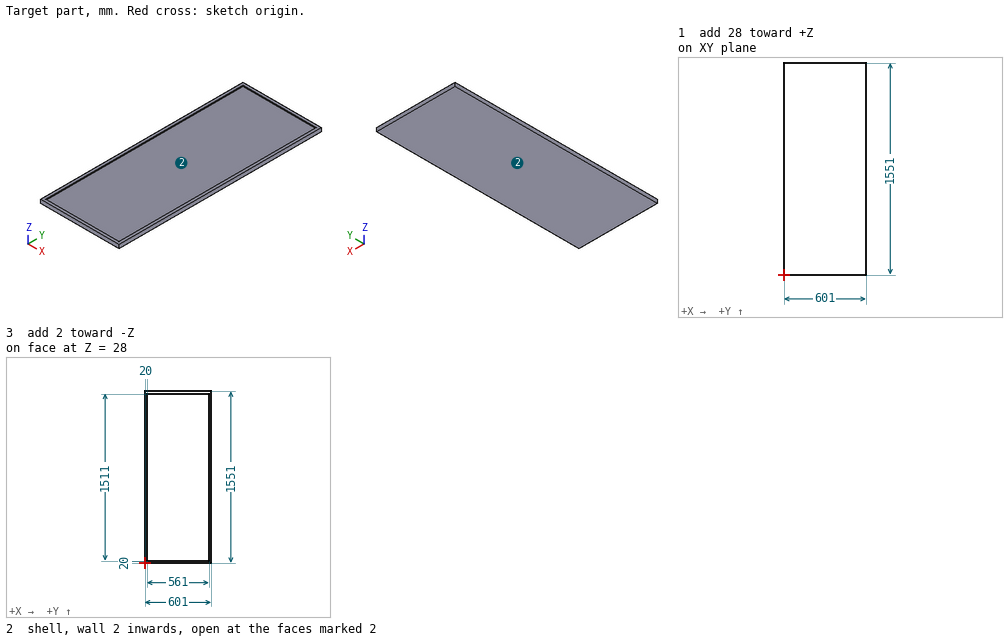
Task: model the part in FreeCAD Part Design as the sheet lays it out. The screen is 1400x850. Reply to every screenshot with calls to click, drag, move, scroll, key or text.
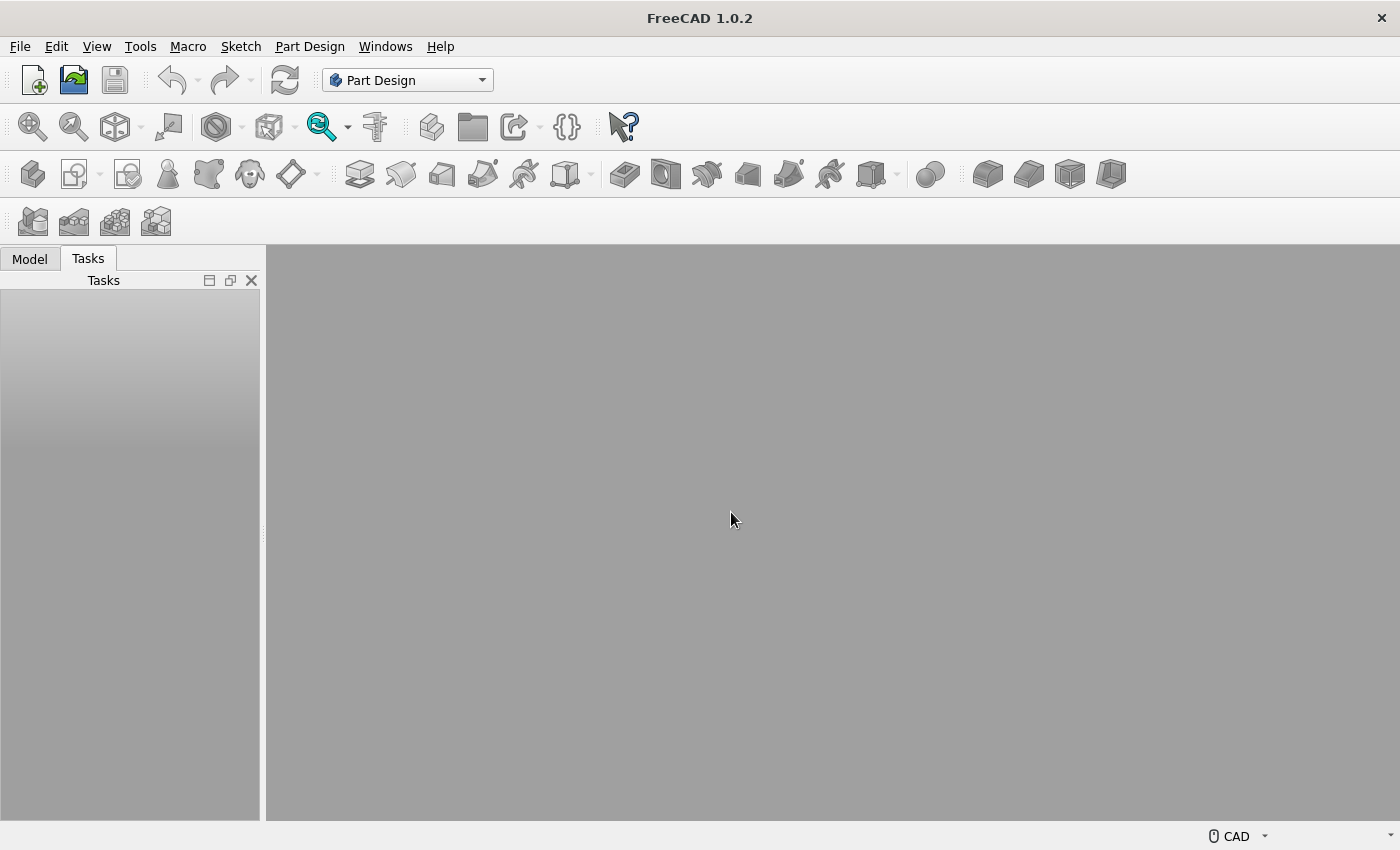
click(33, 80)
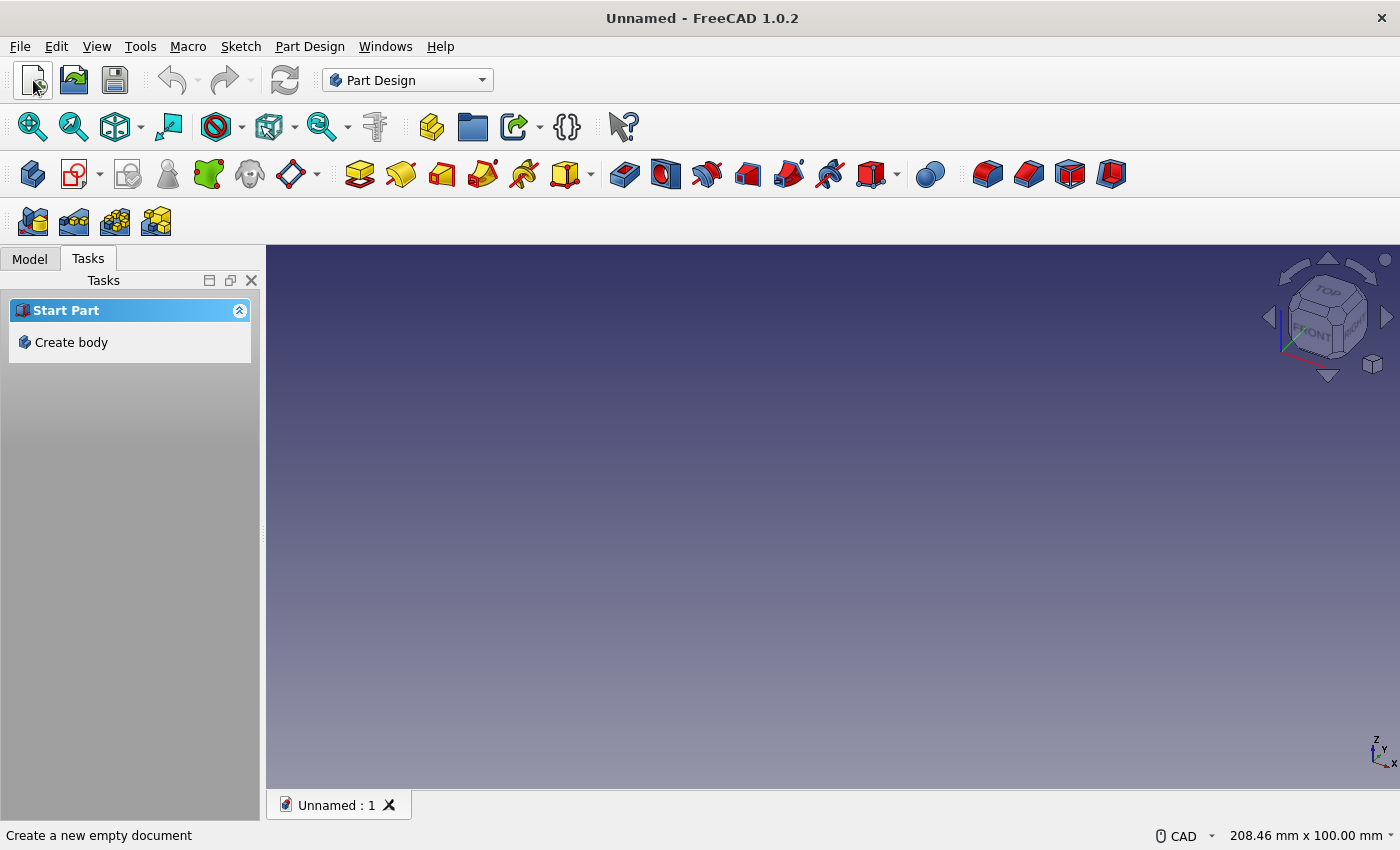
click(74, 174)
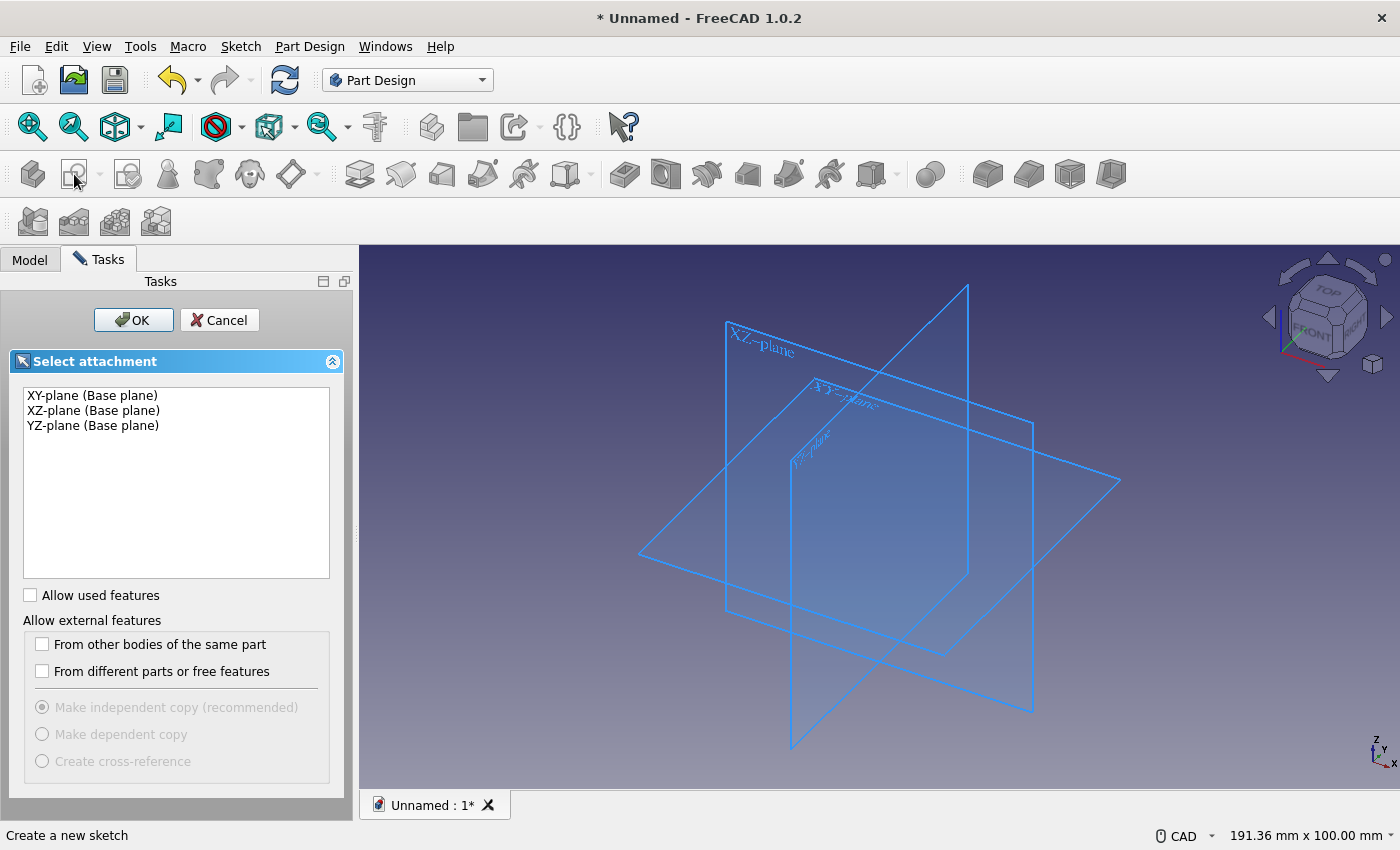
click(84, 396)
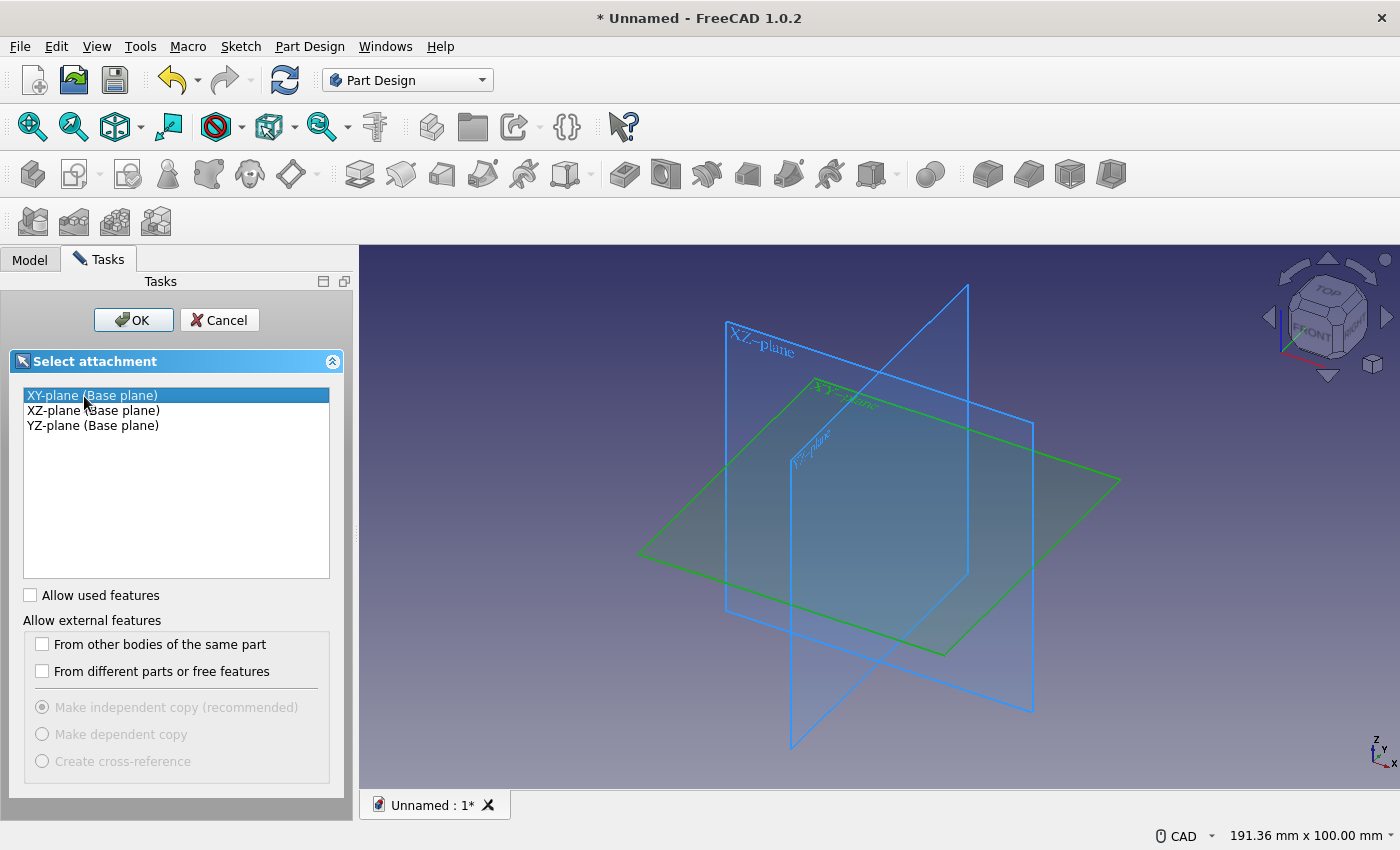
click(134, 320)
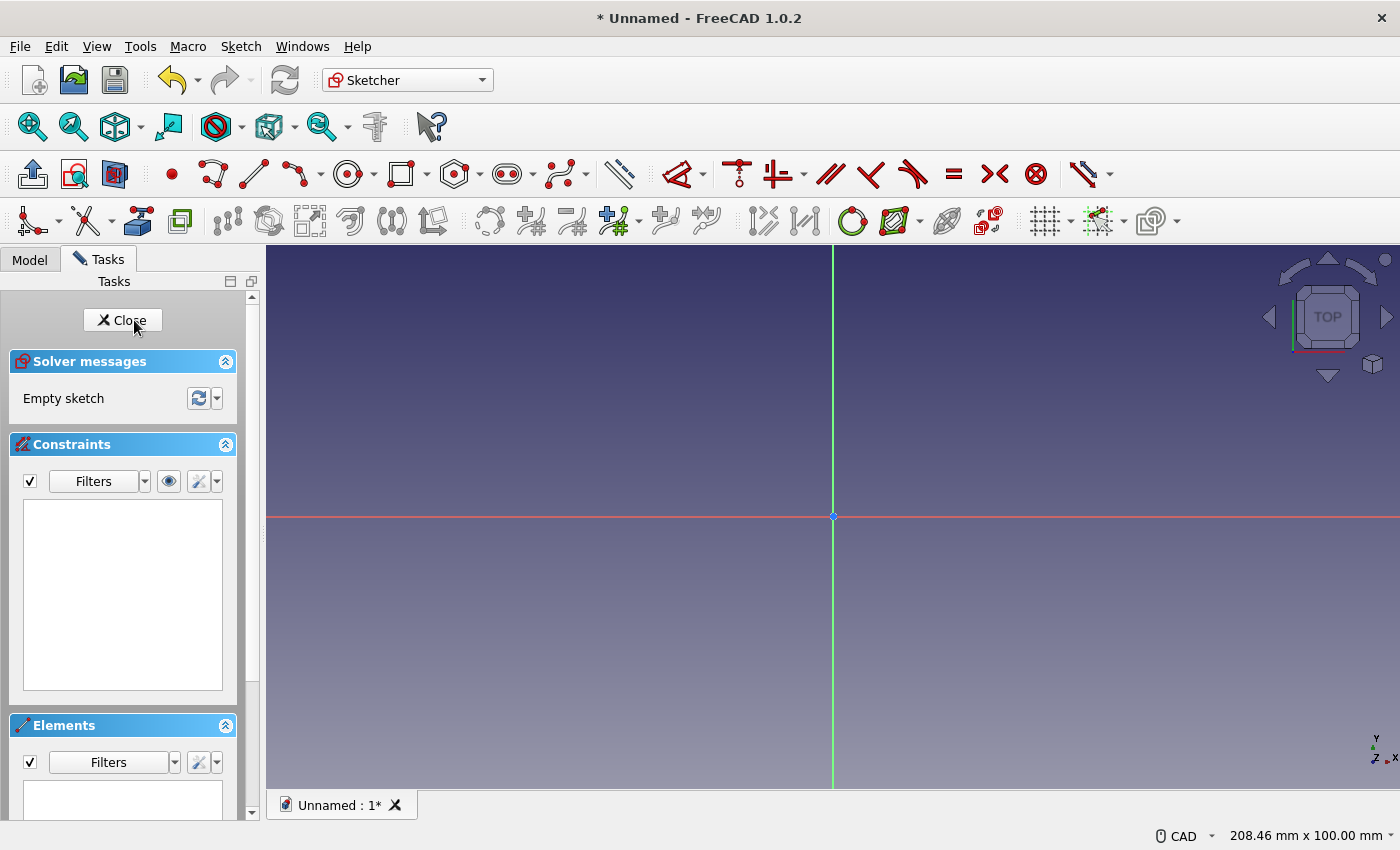
scroll(675, 738, down, 15)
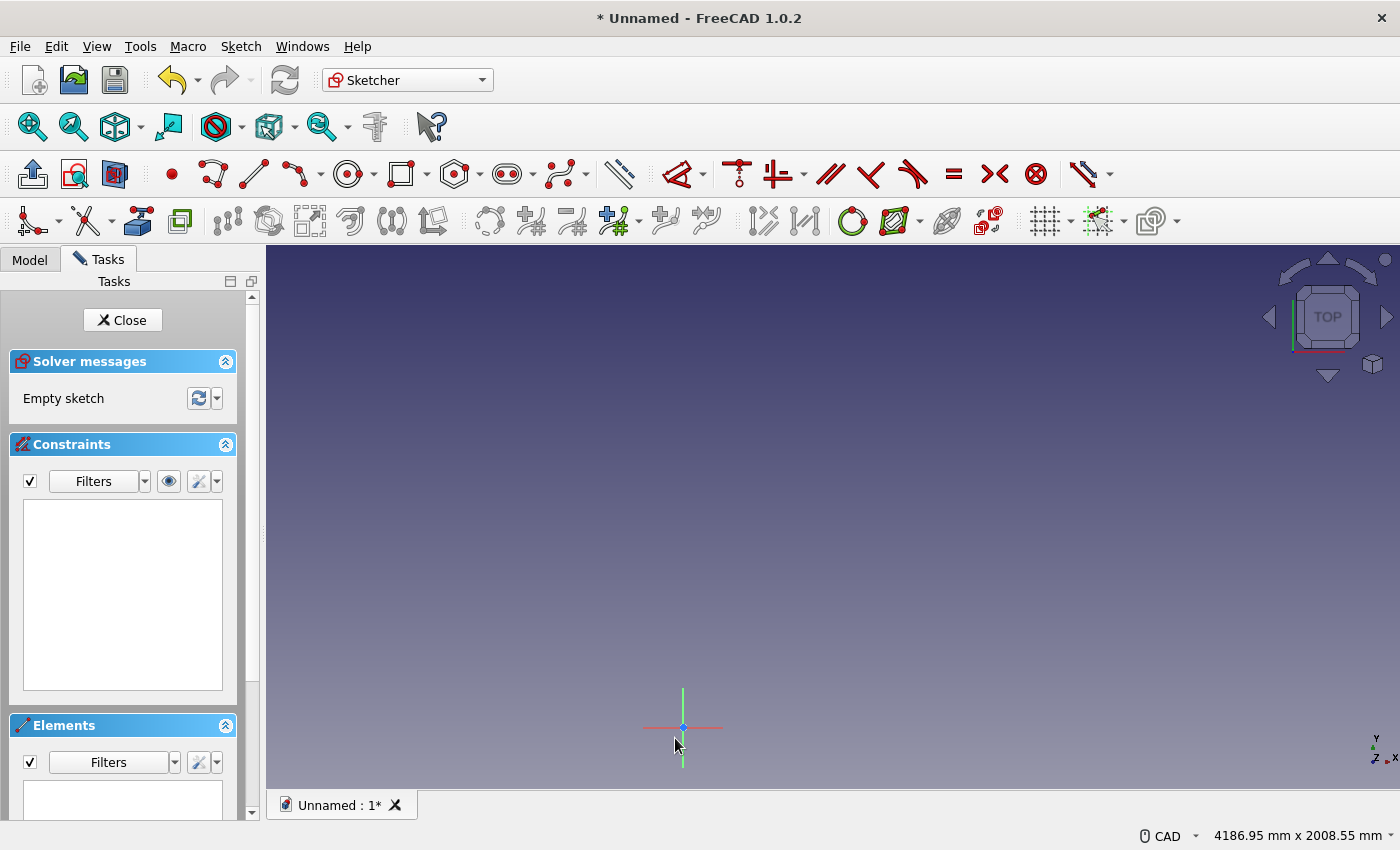
click(400, 174)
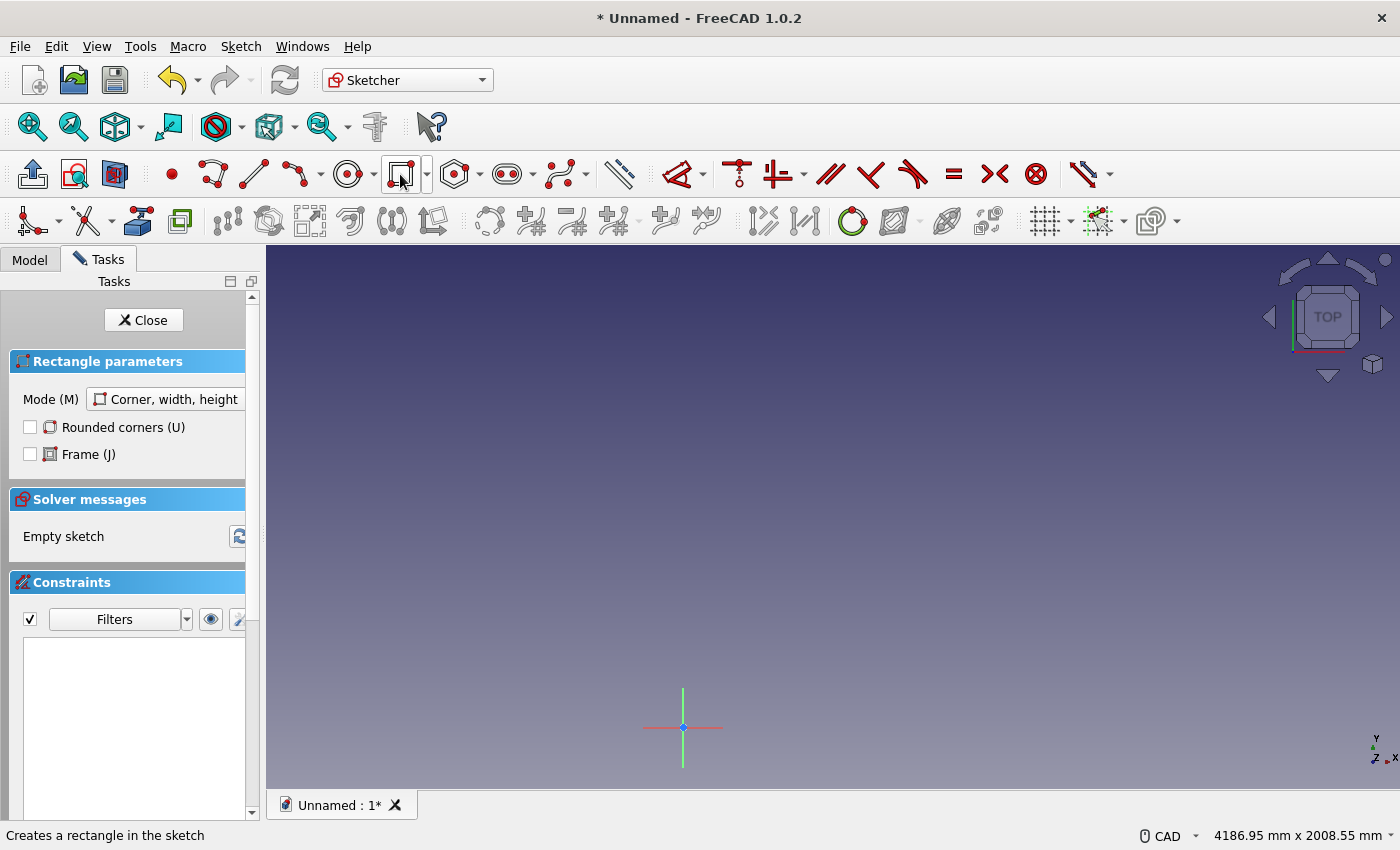
click(683, 728)
click(846, 308)
key(Escape)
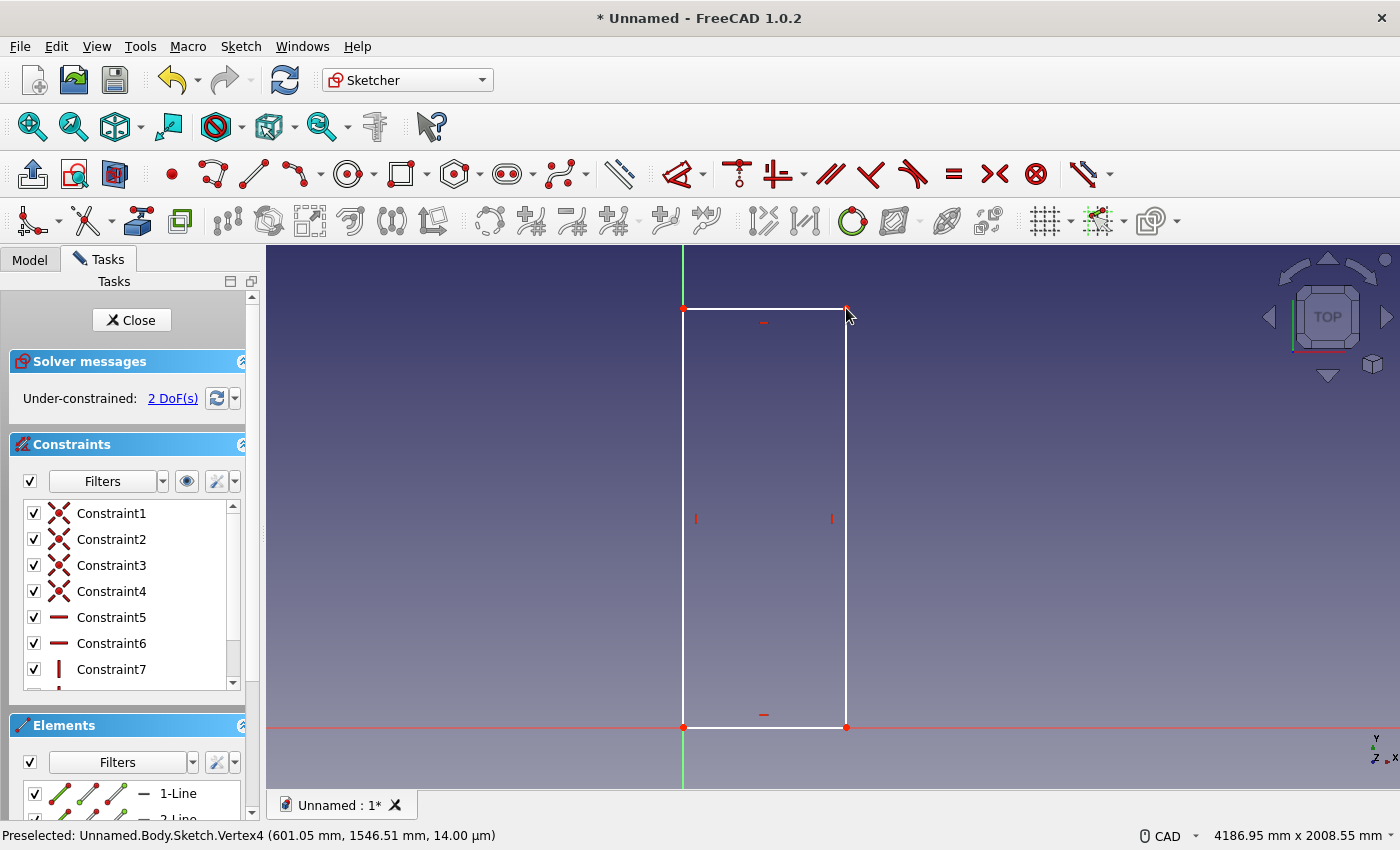
click(676, 174)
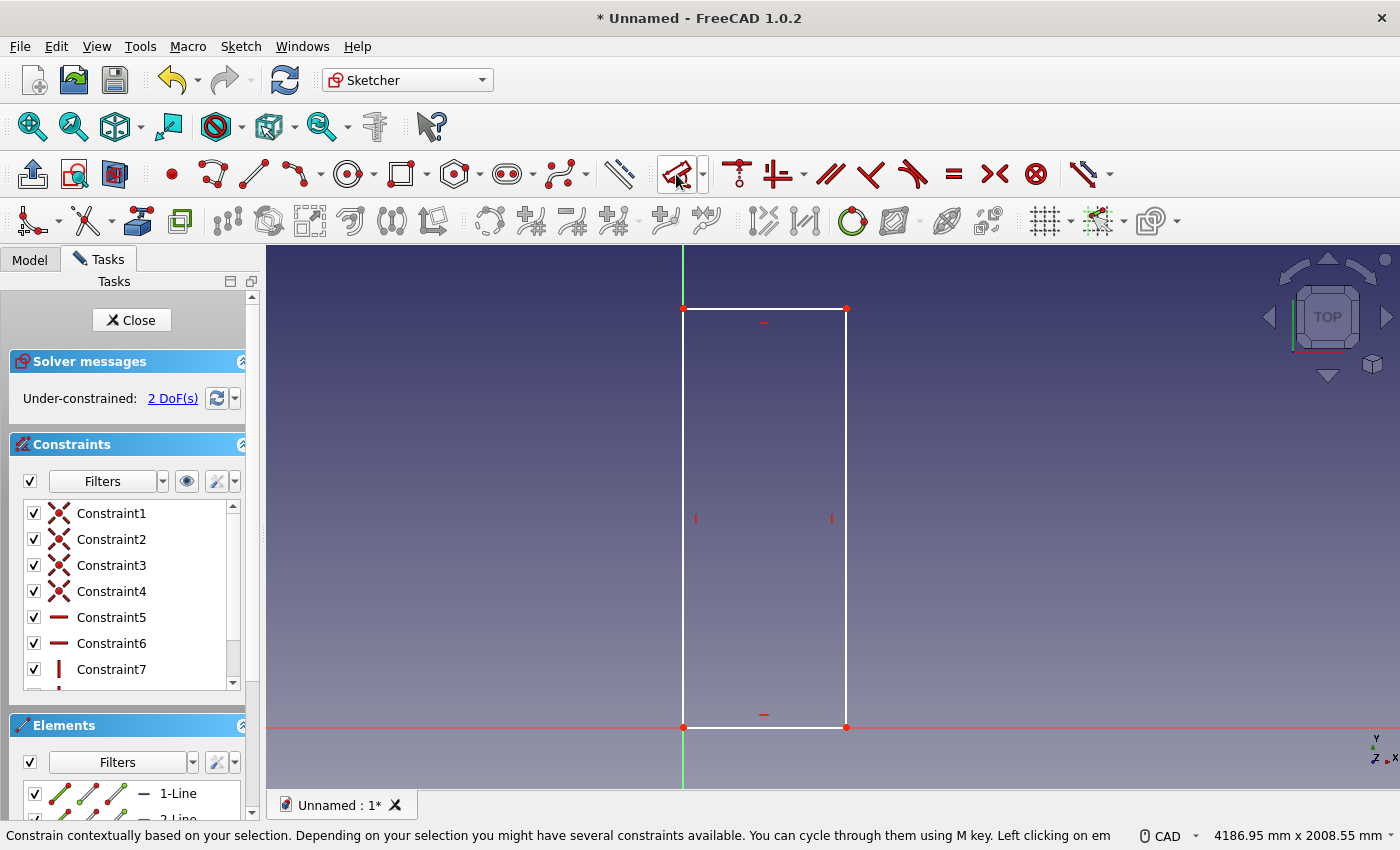
click(732, 728)
click(765, 694)